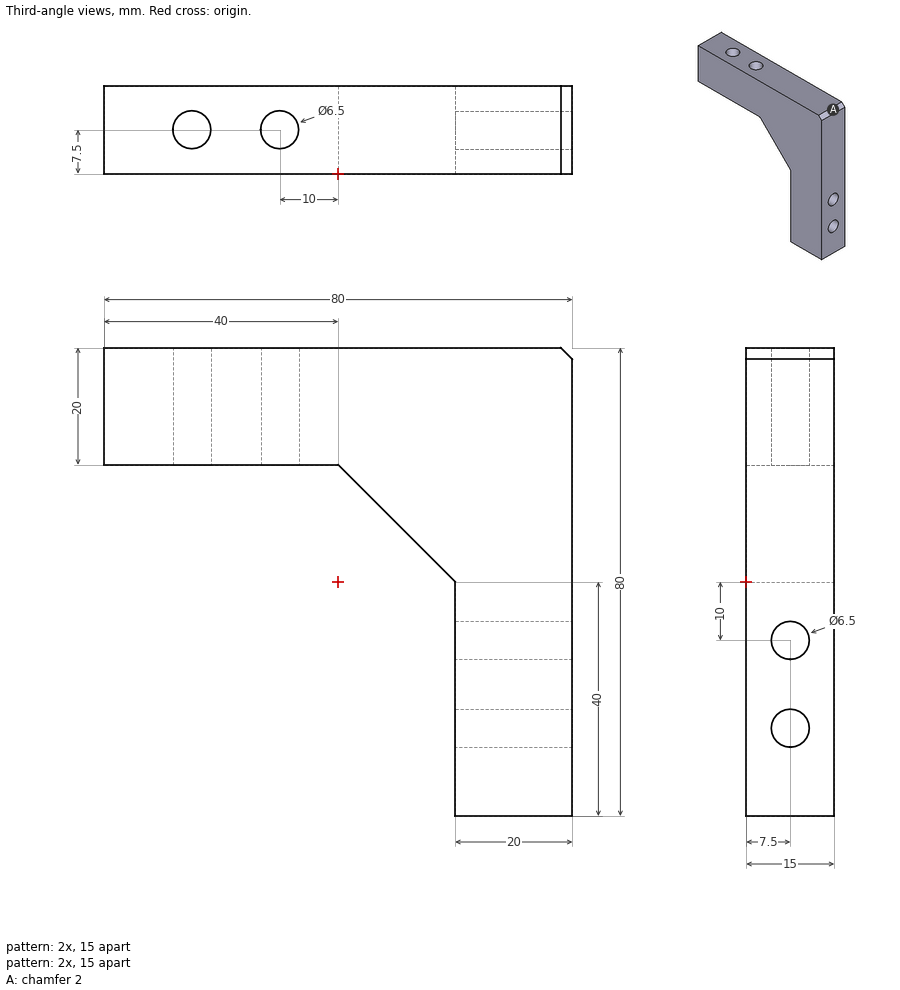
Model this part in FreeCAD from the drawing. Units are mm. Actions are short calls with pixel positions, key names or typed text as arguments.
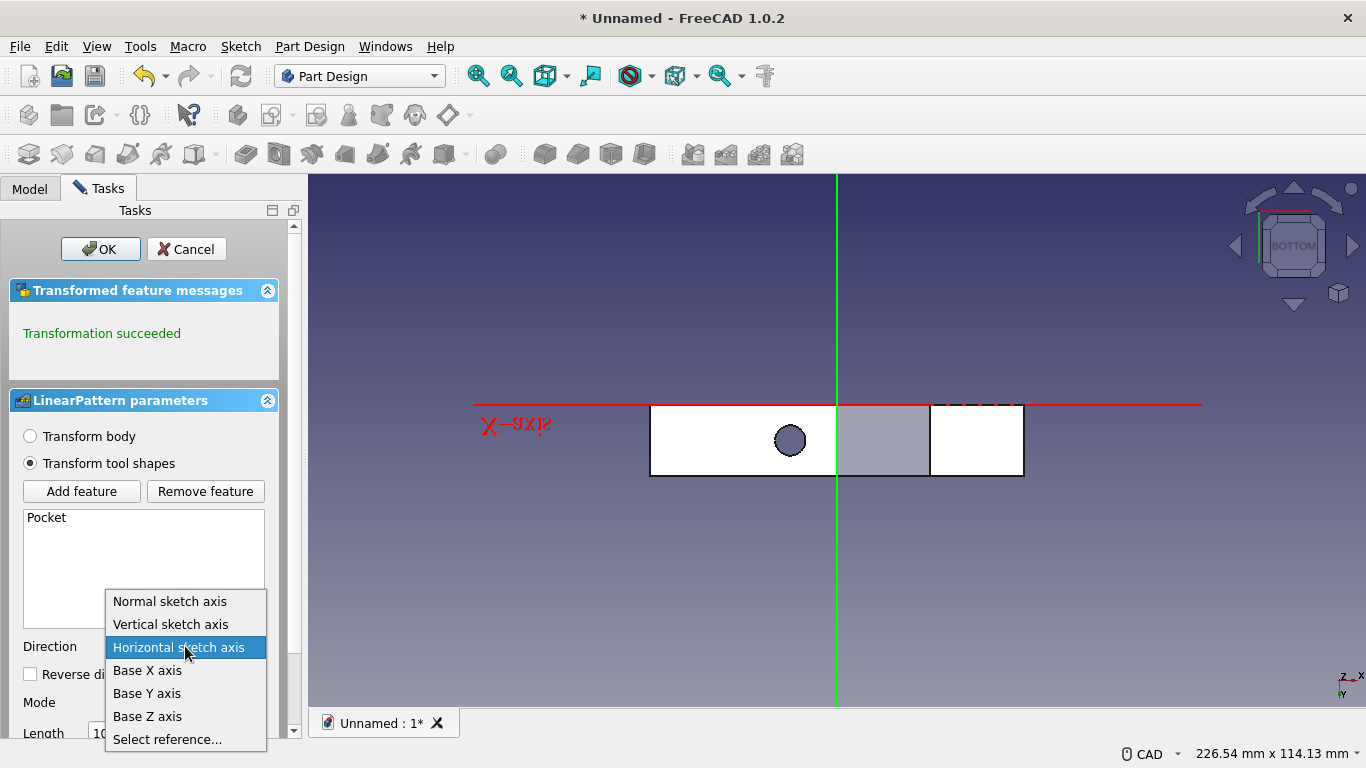
click(184, 670)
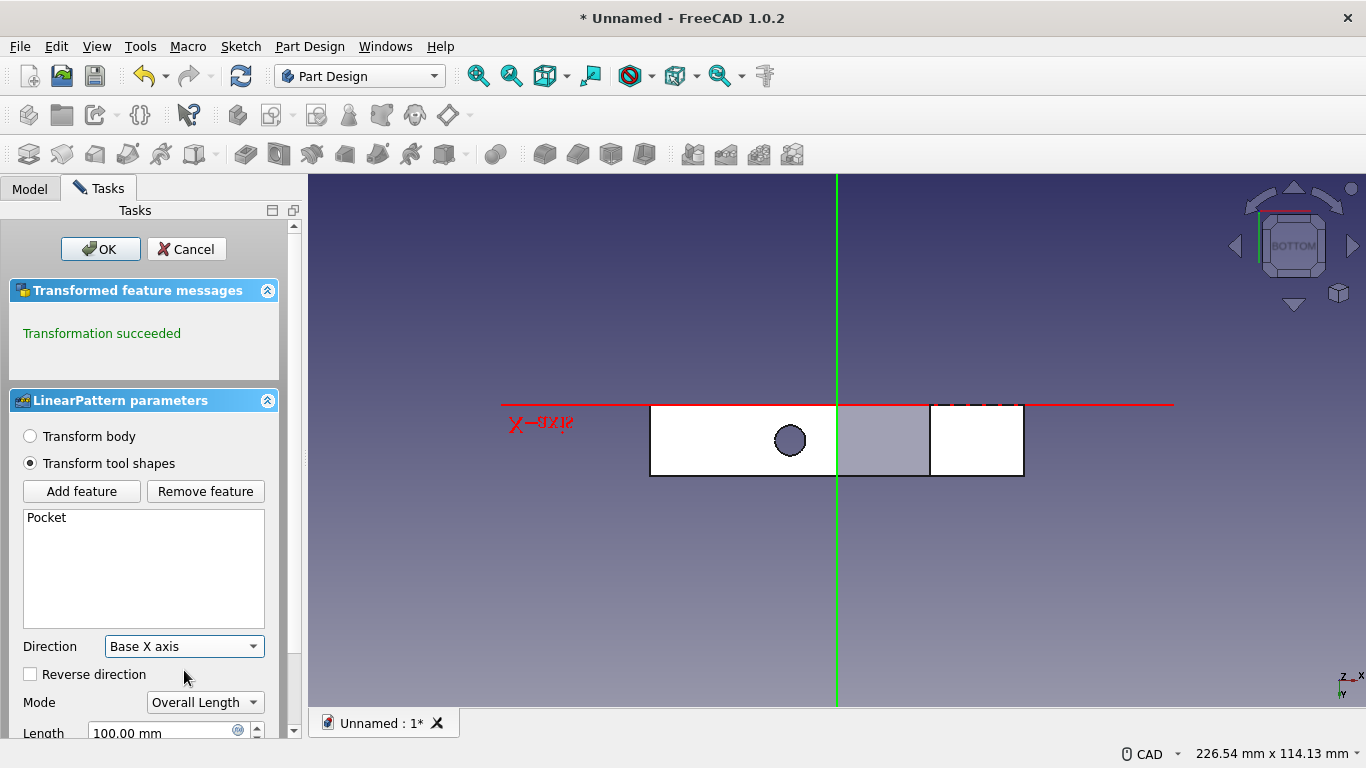
click(206, 702)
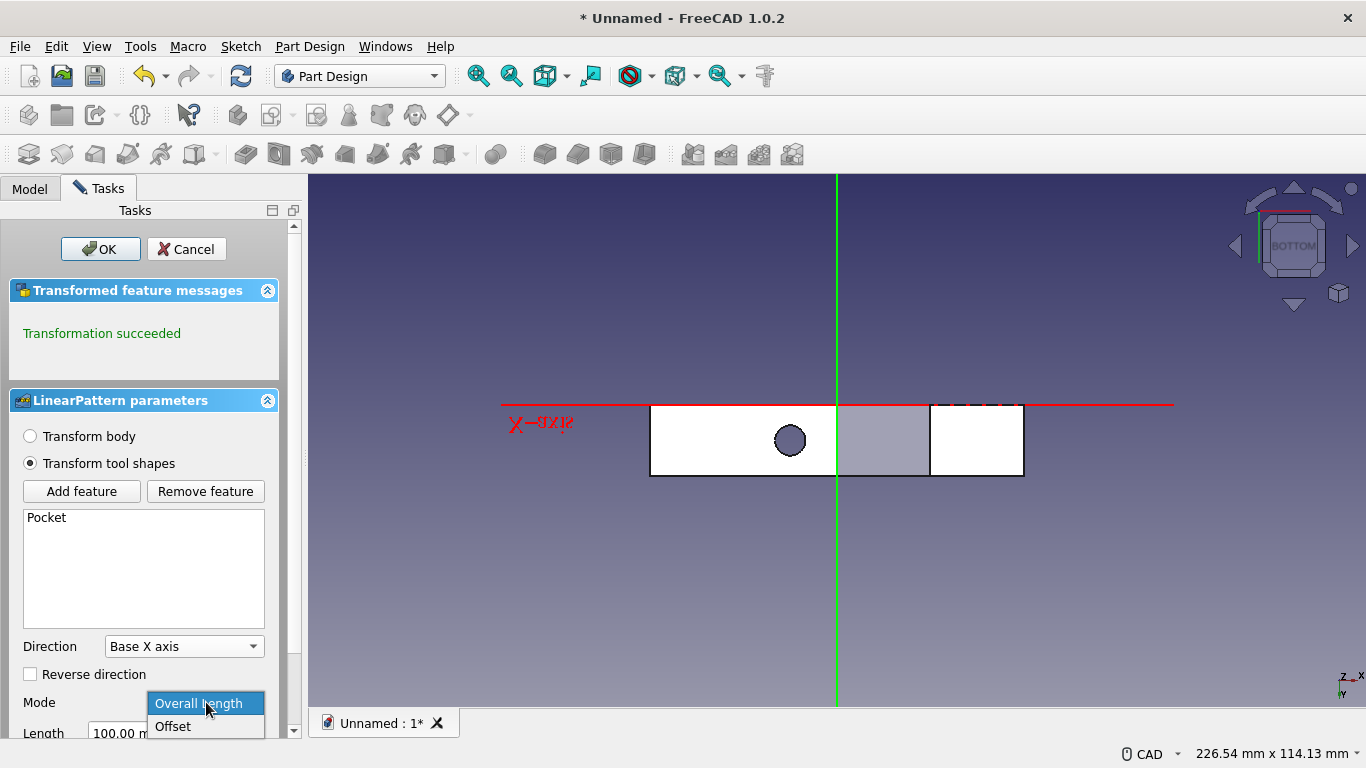
click(204, 726)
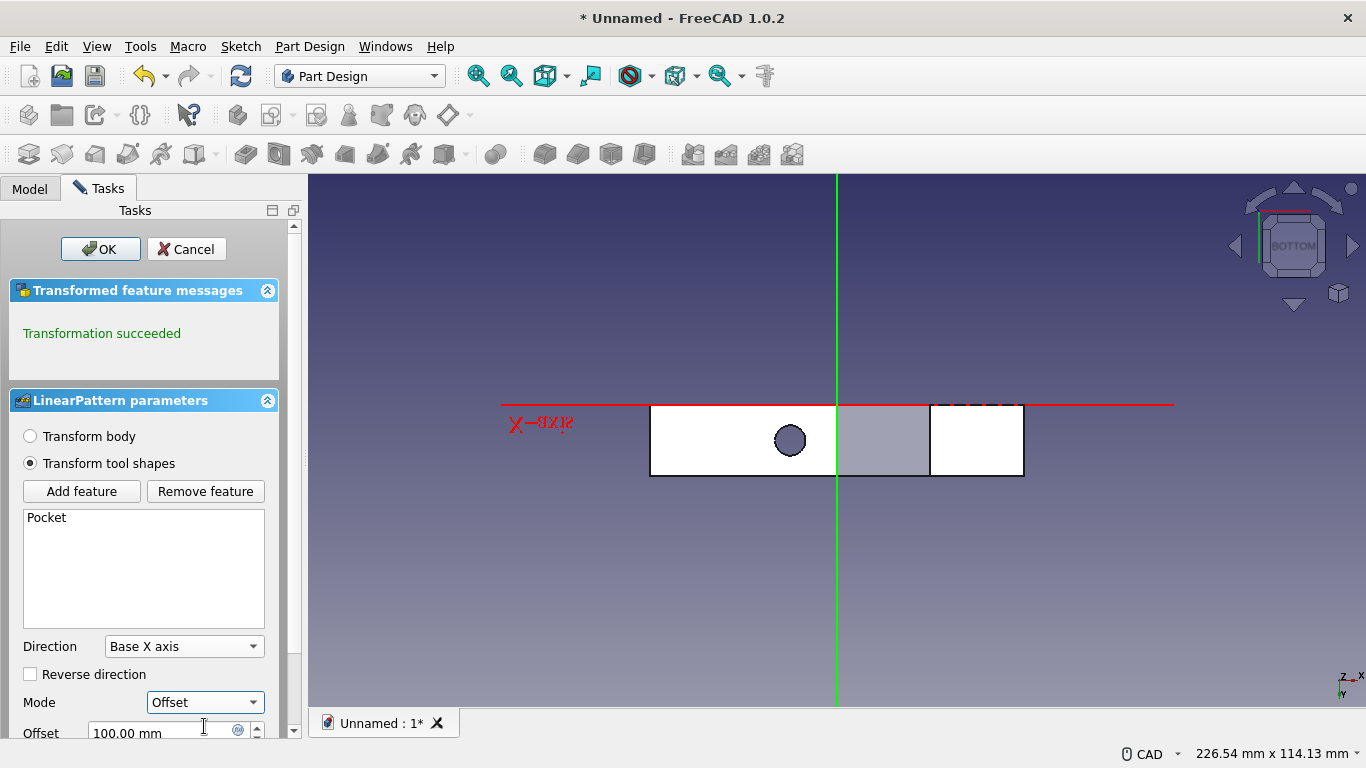
scroll(294, 479, down, 2)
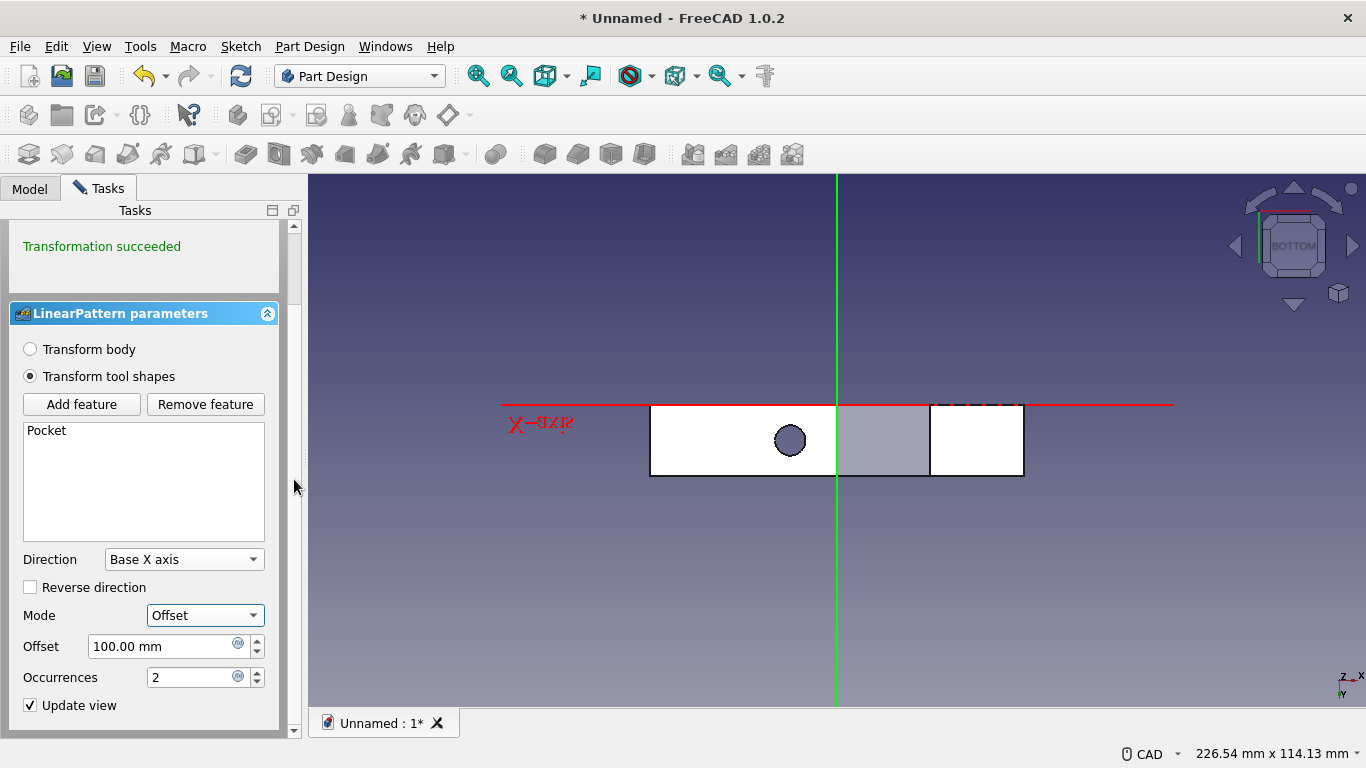
triple_click(170, 646)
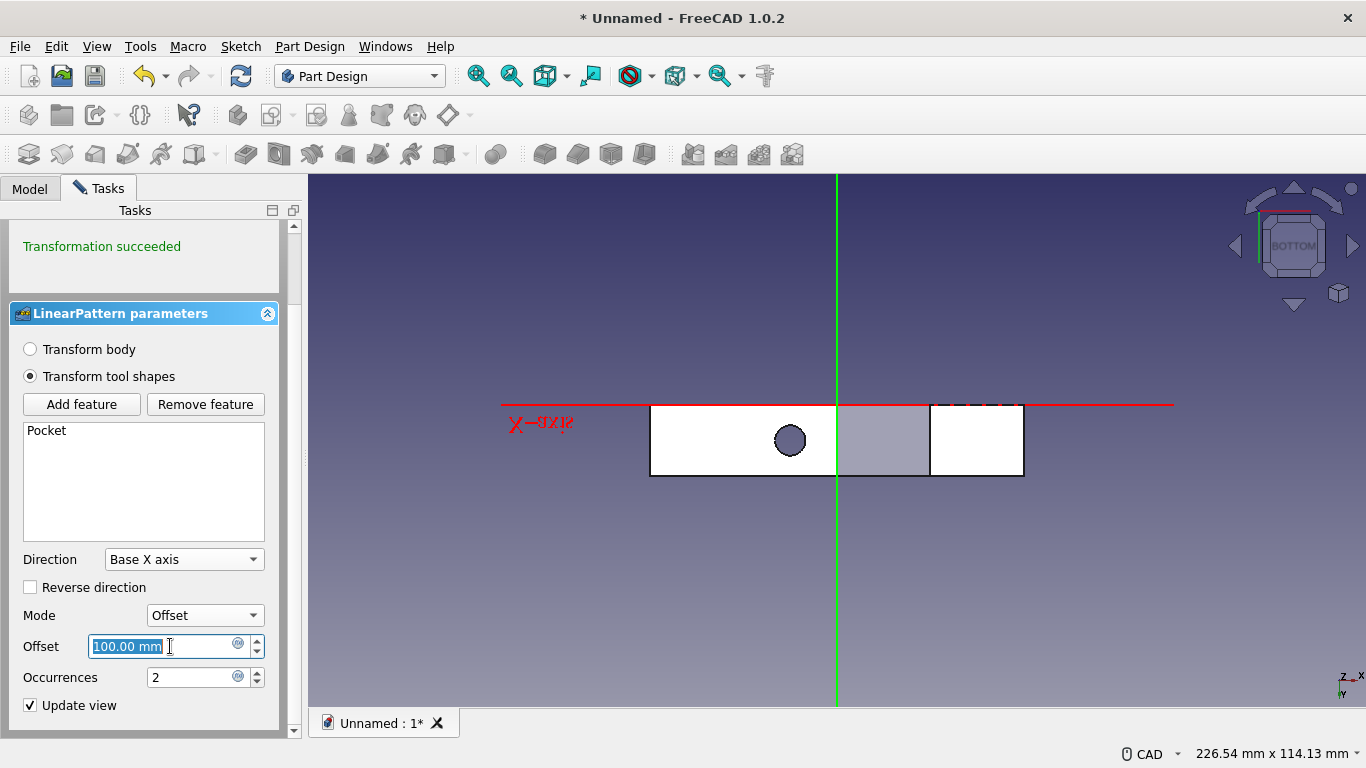
text(15)
key(Tab)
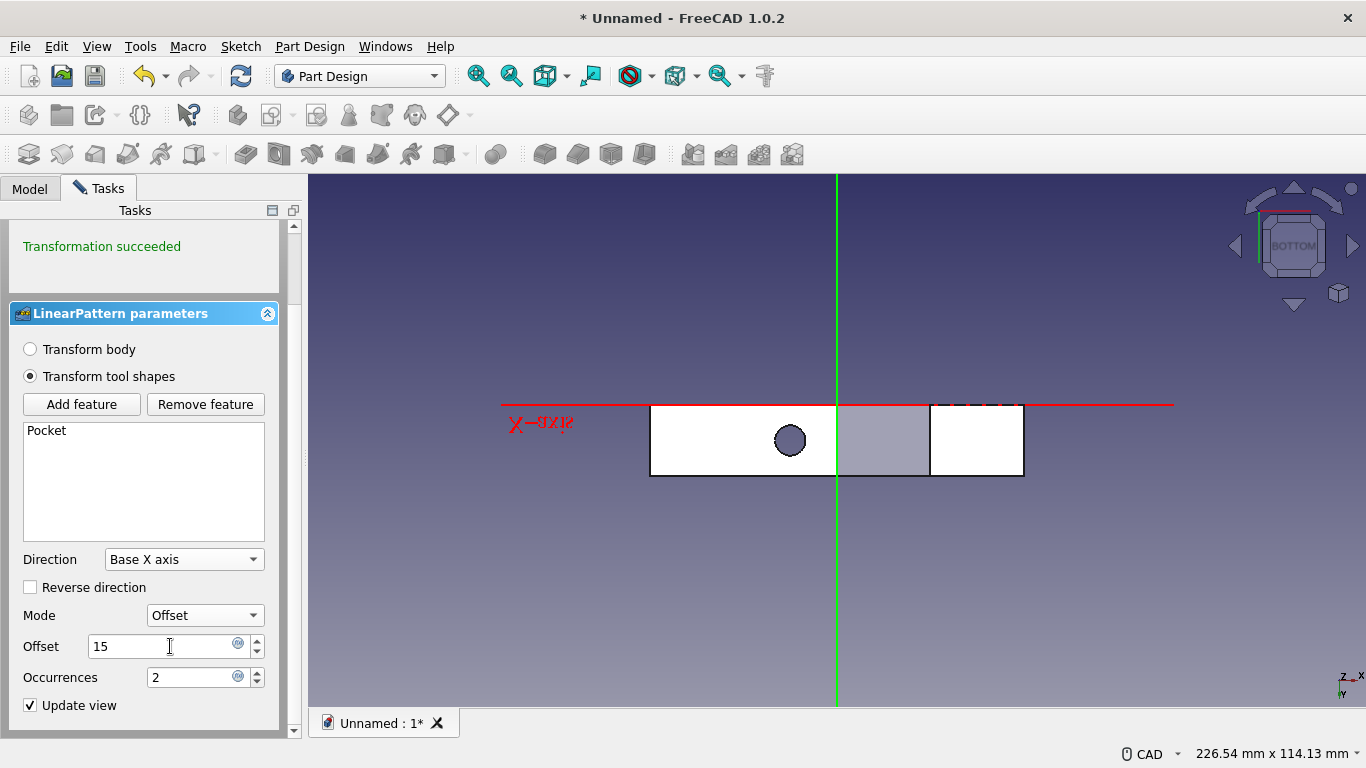
triple_click(199, 678)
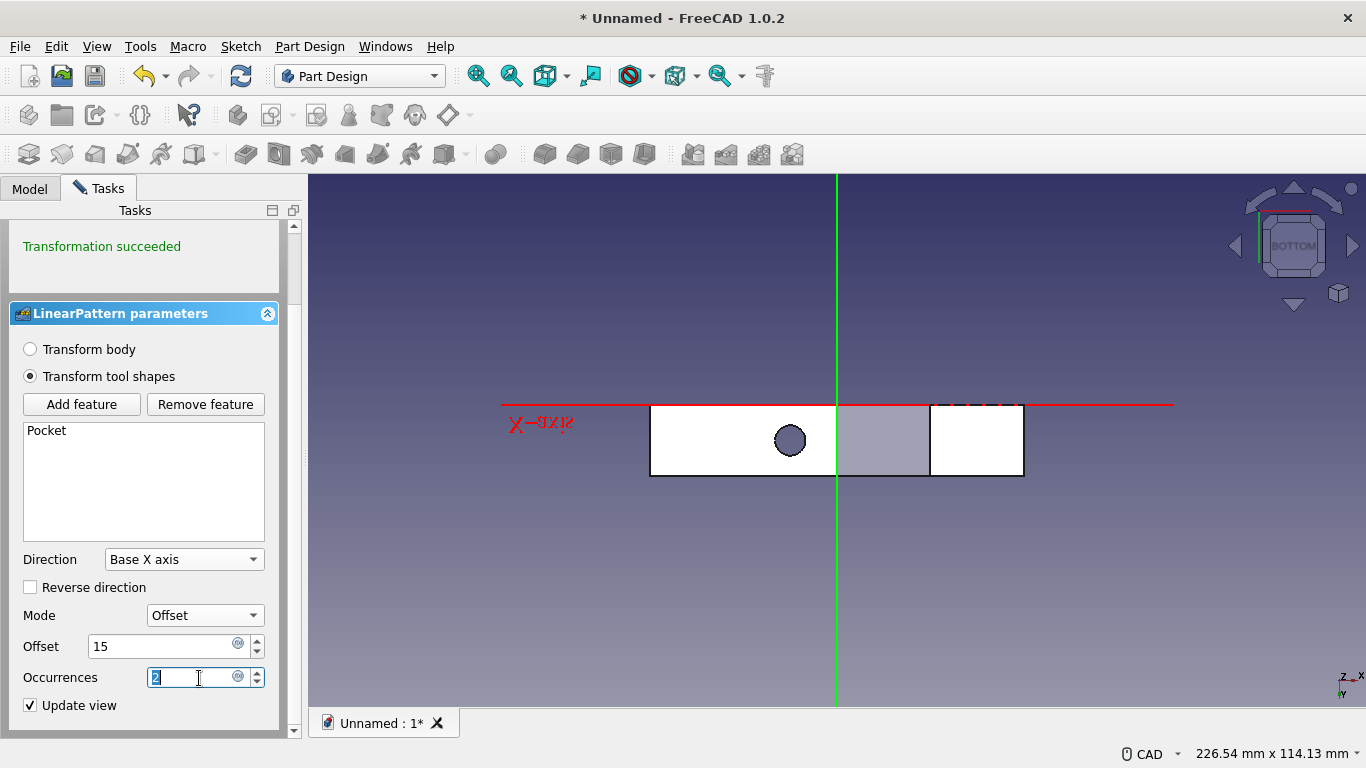
text(2)
key(Tab)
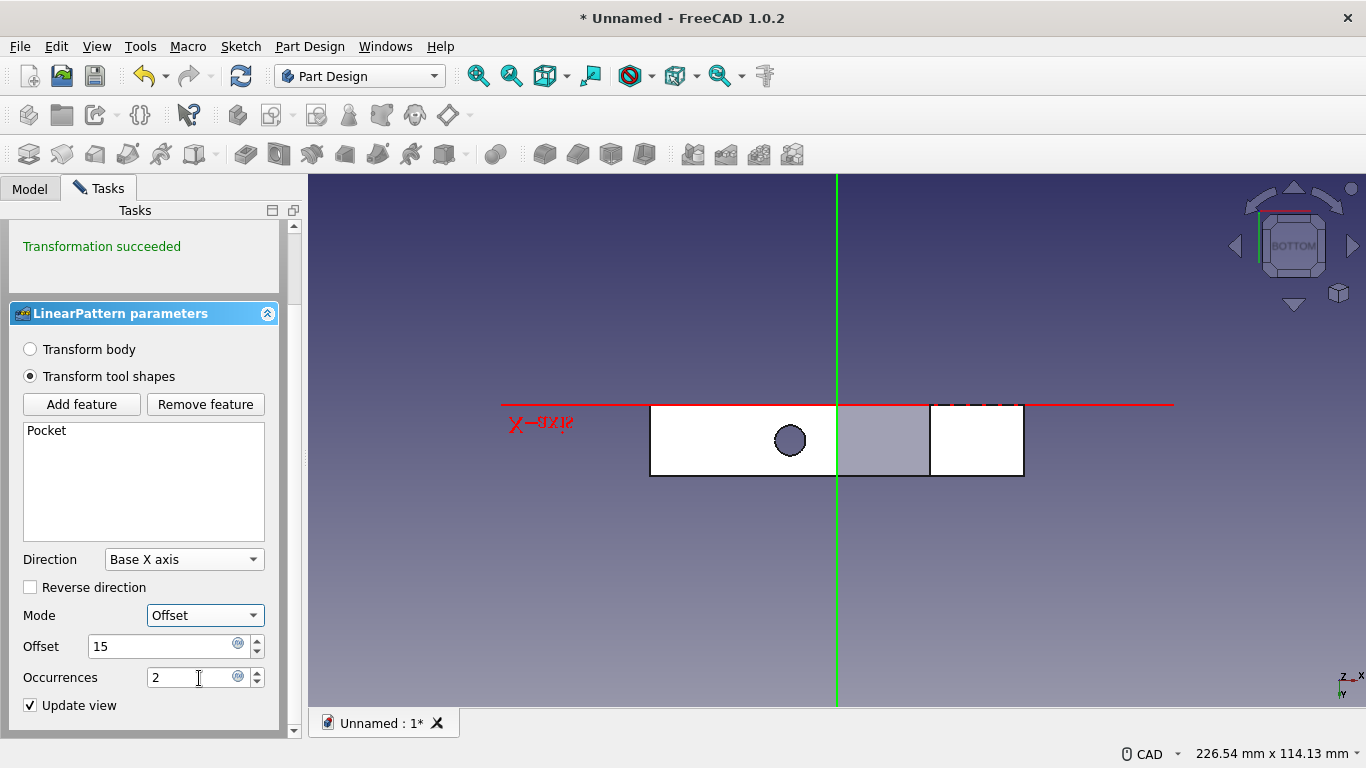
click(31, 587)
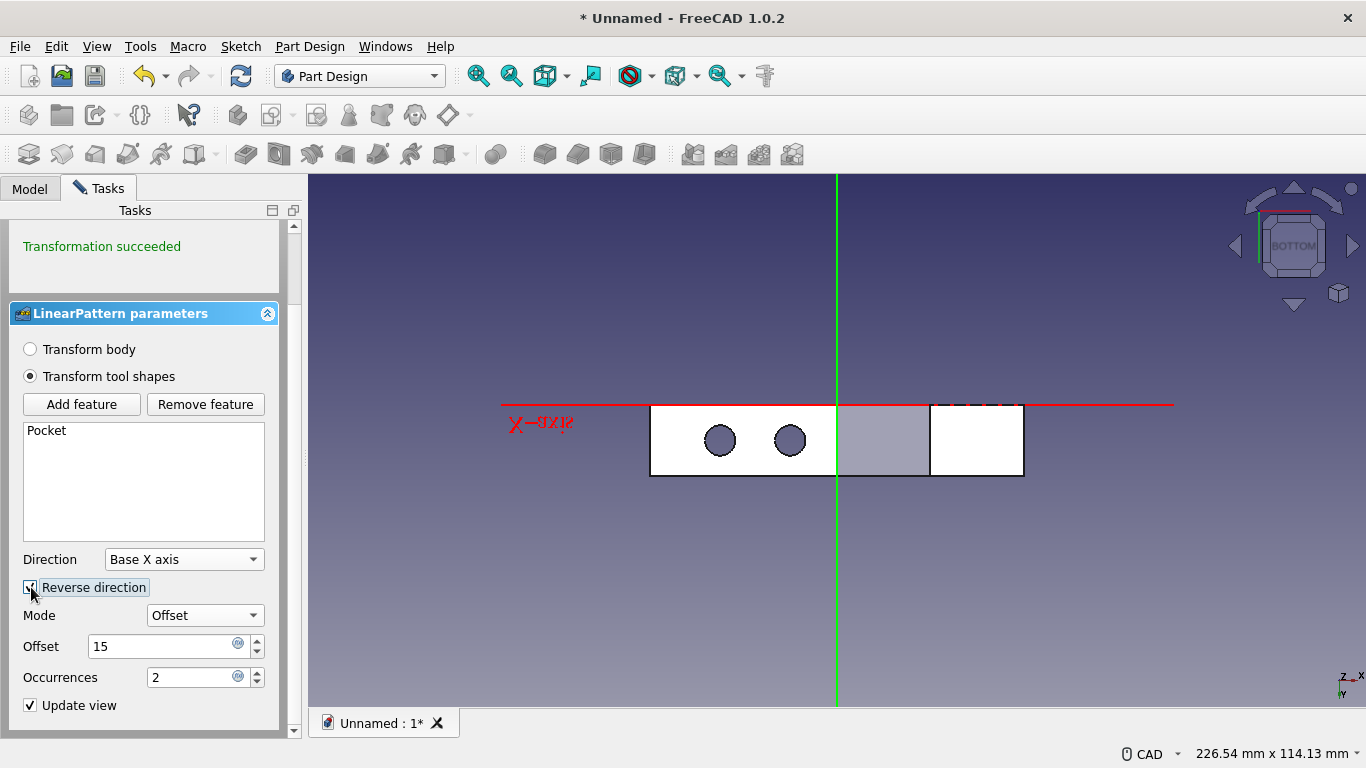
scroll(294, 479, up, 3)